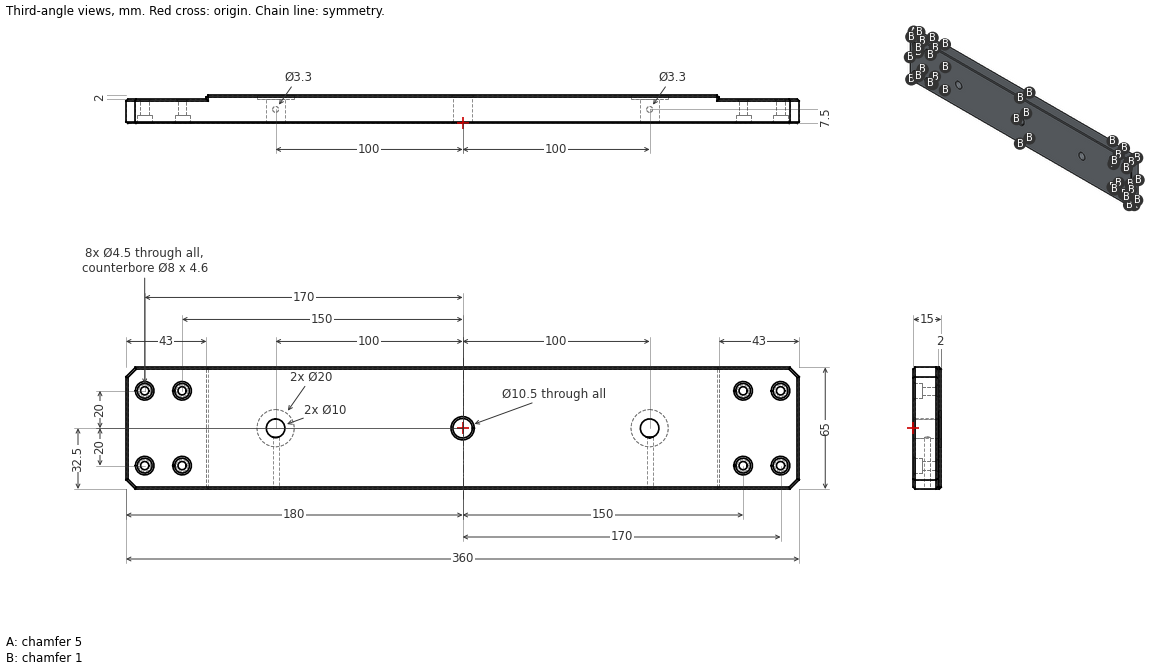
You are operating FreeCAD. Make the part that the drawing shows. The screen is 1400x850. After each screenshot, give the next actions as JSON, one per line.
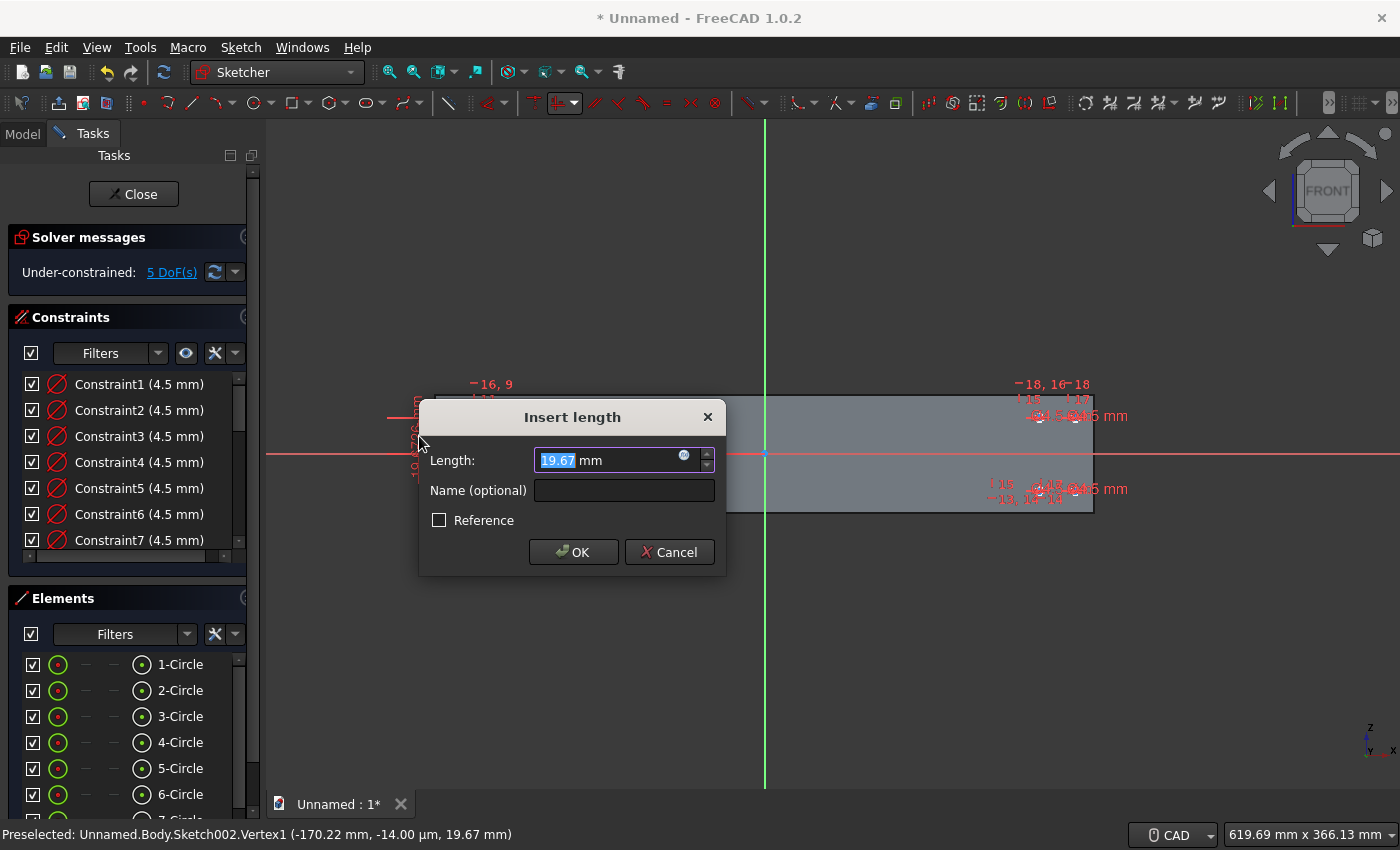
{"action": "type", "text": "20"}
{"action": "key", "text": "Return"}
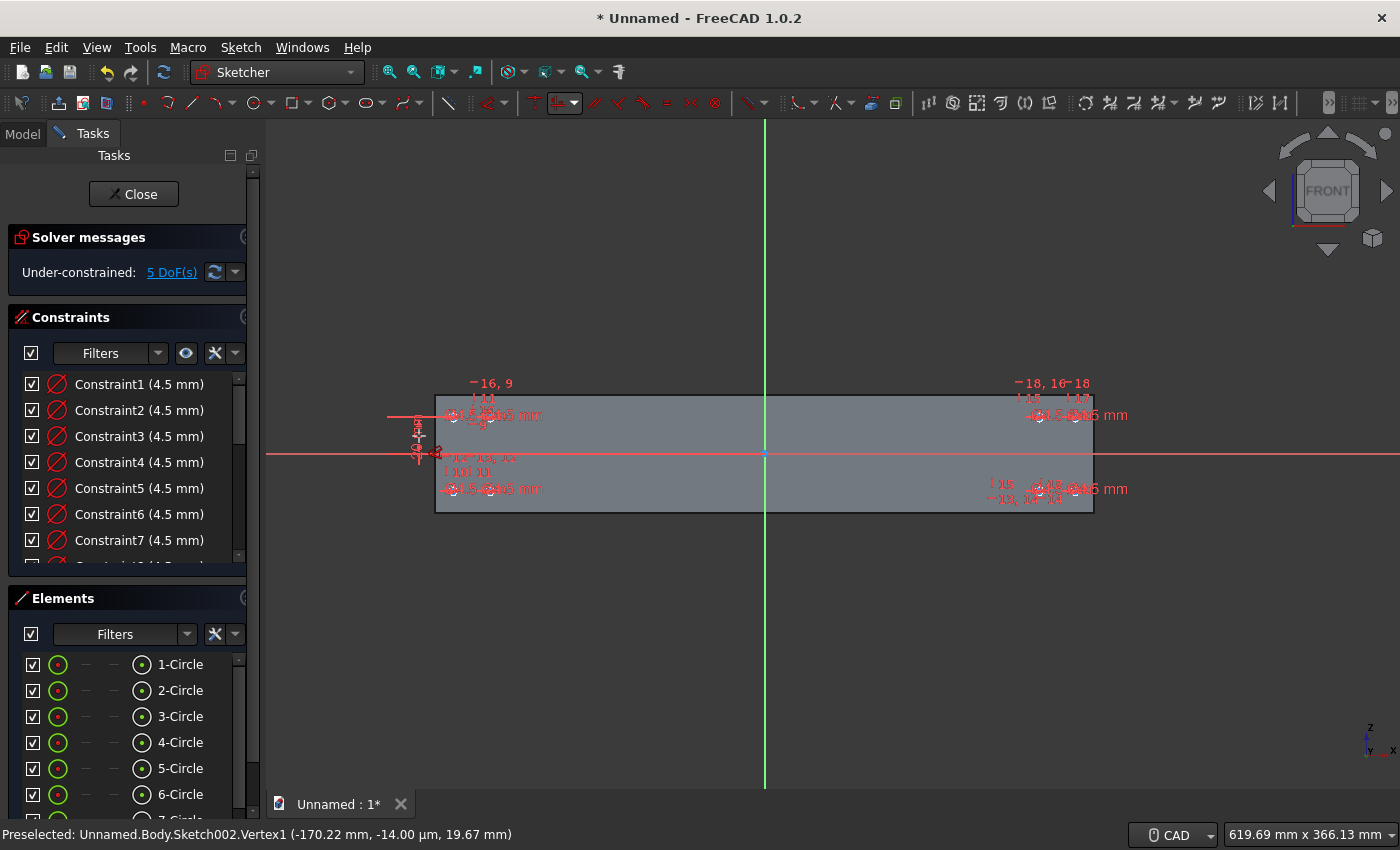
{"action": "left_click", "coordinate": [453, 491]}
{"action": "left_click", "coordinate": [419, 473]}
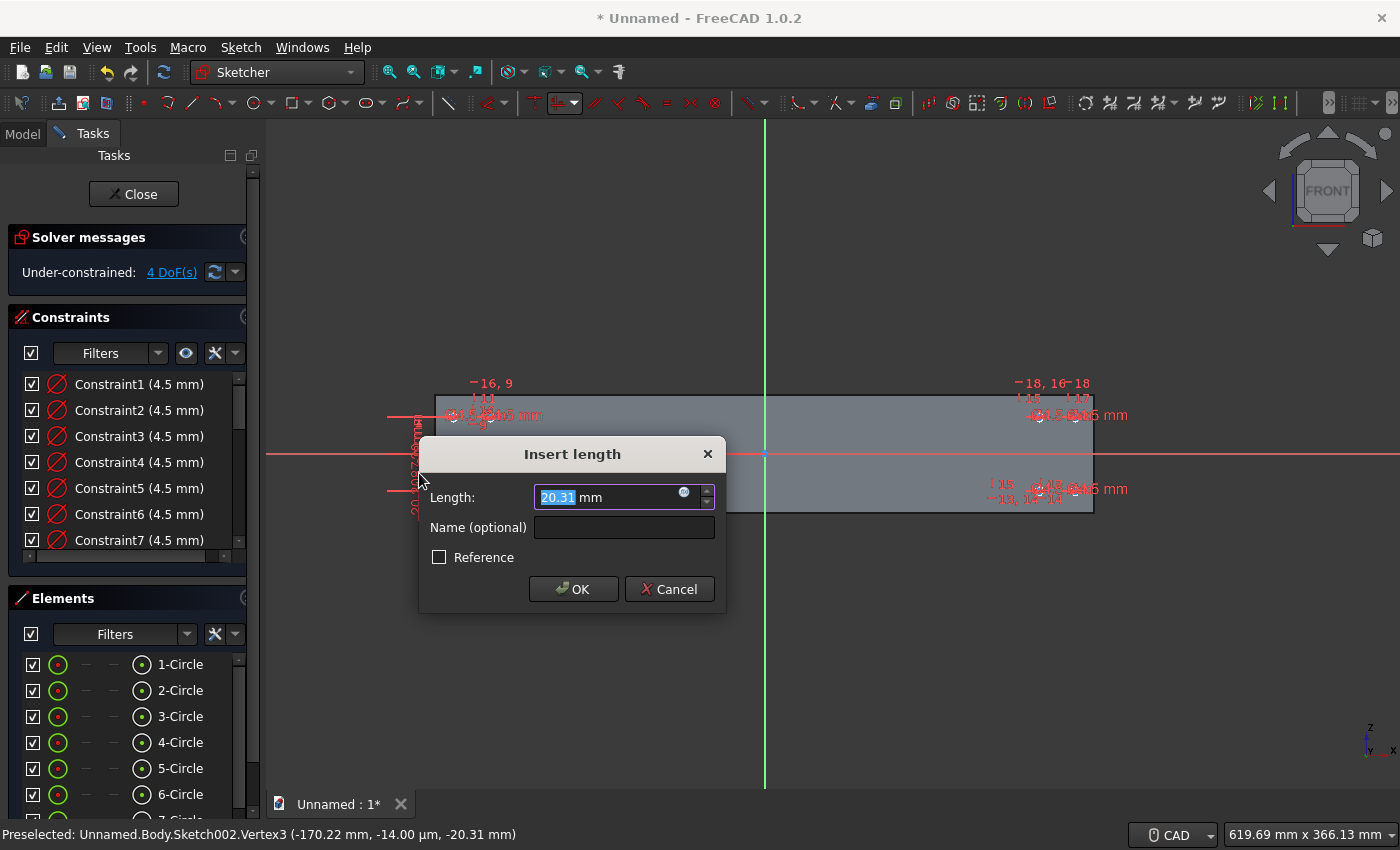
{"action": "type", "text": "20"}
{"action": "key", "text": "Return"}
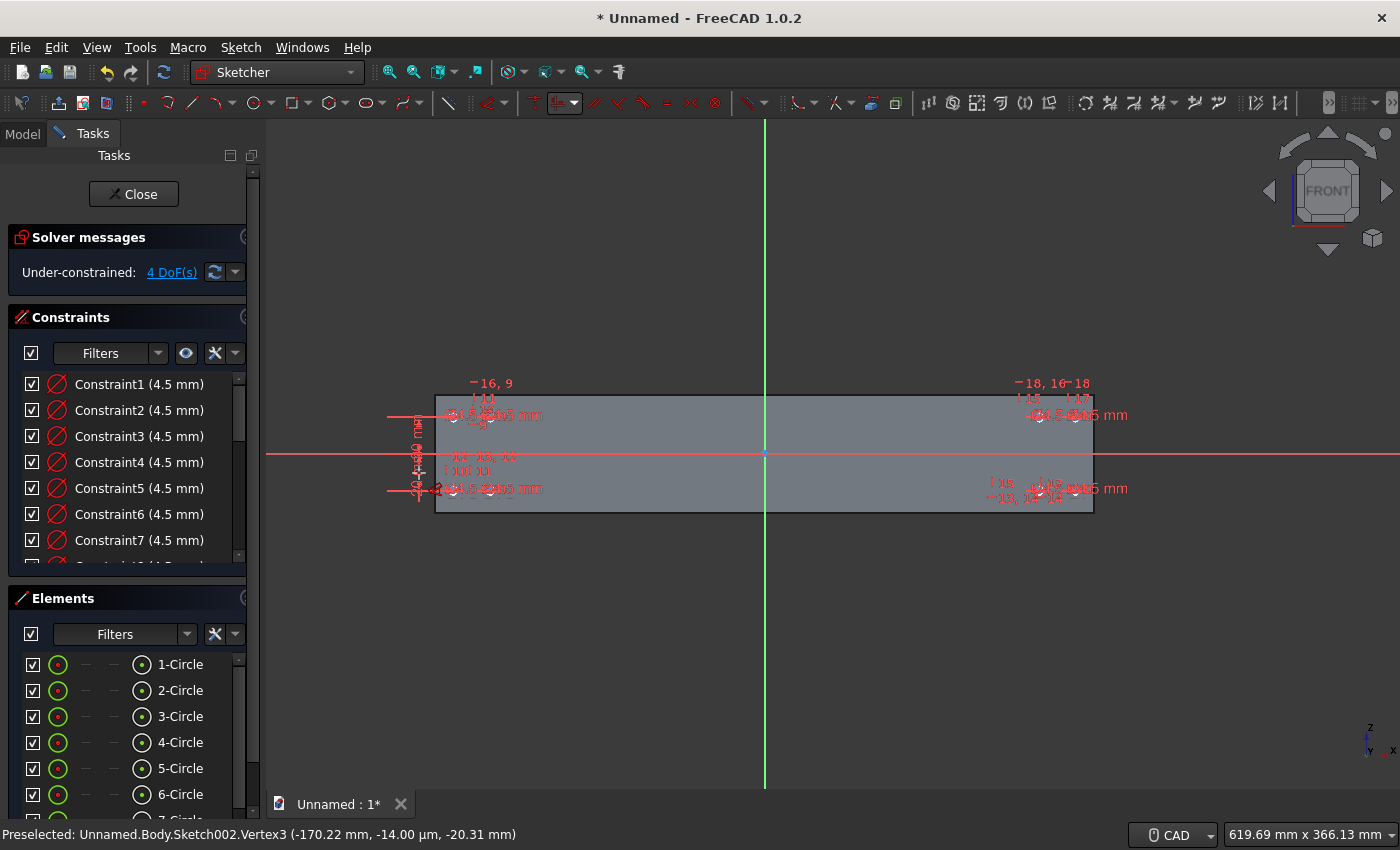
{"action": "left_click", "coordinate": [453, 417]}
{"action": "left_click", "coordinate": [609, 383]}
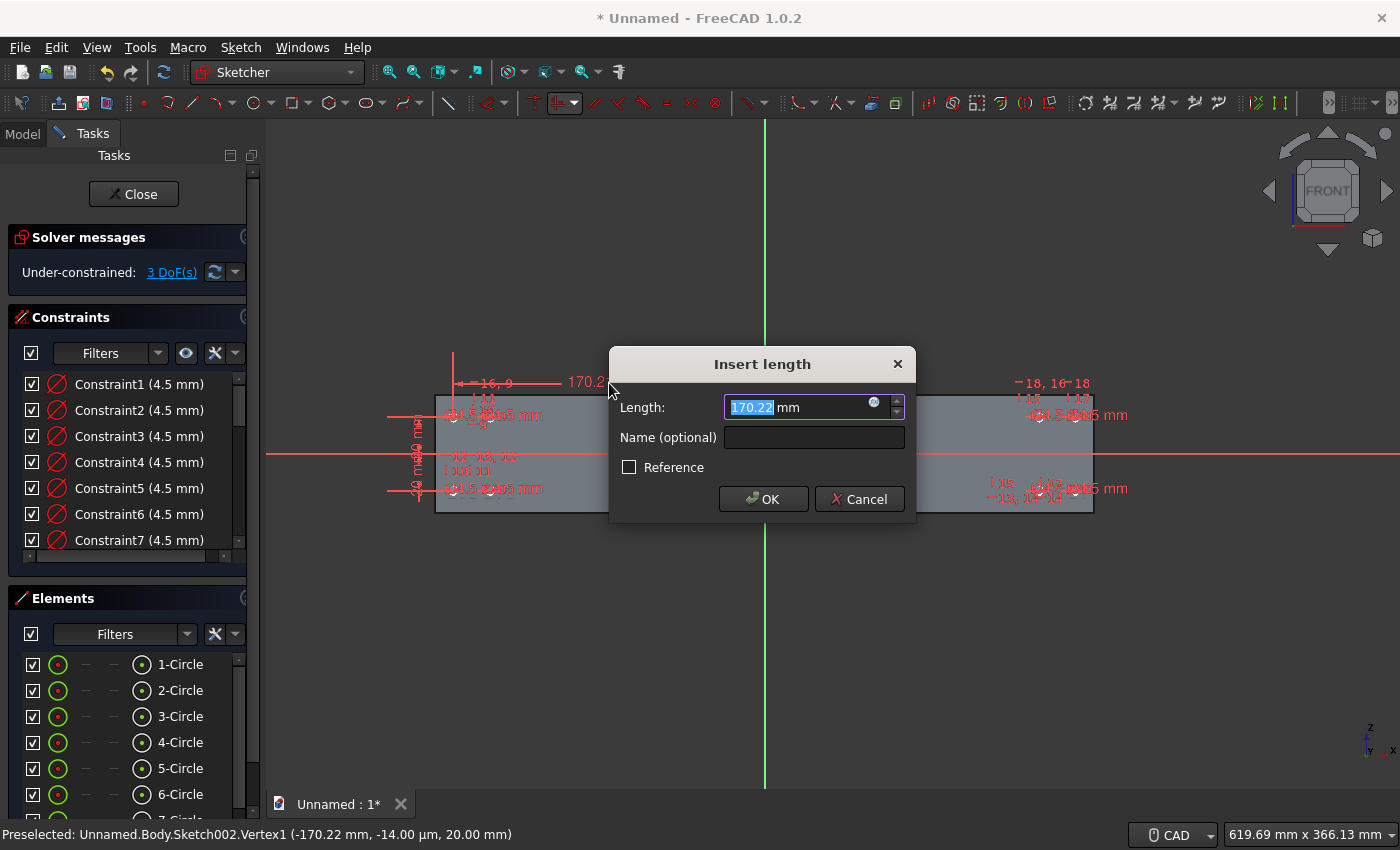
{"action": "type", "text": "170"}
{"action": "key", "text": "Return"}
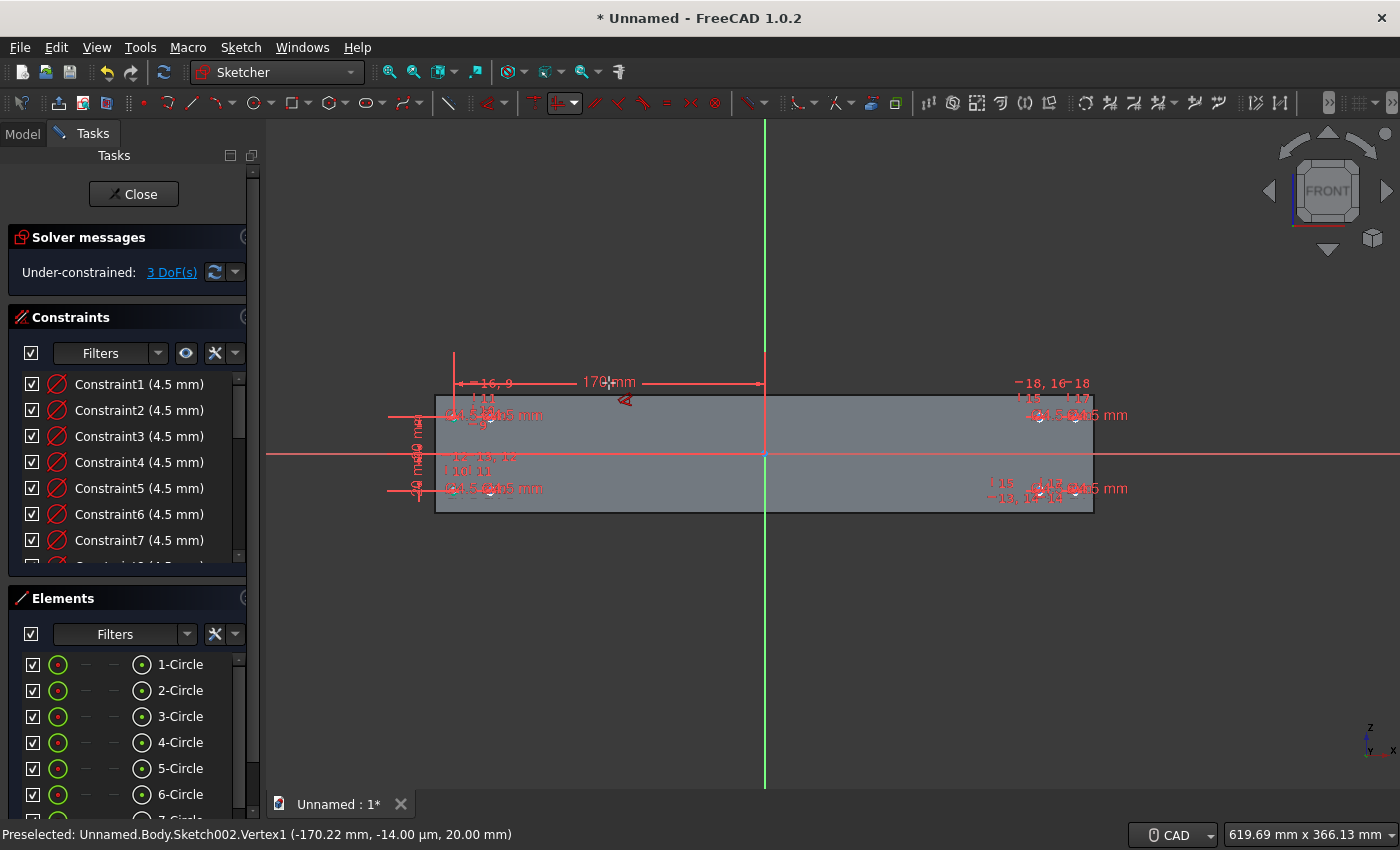
{"action": "left_click", "coordinate": [490, 417]}
{"action": "left_click", "coordinate": [691, 383]}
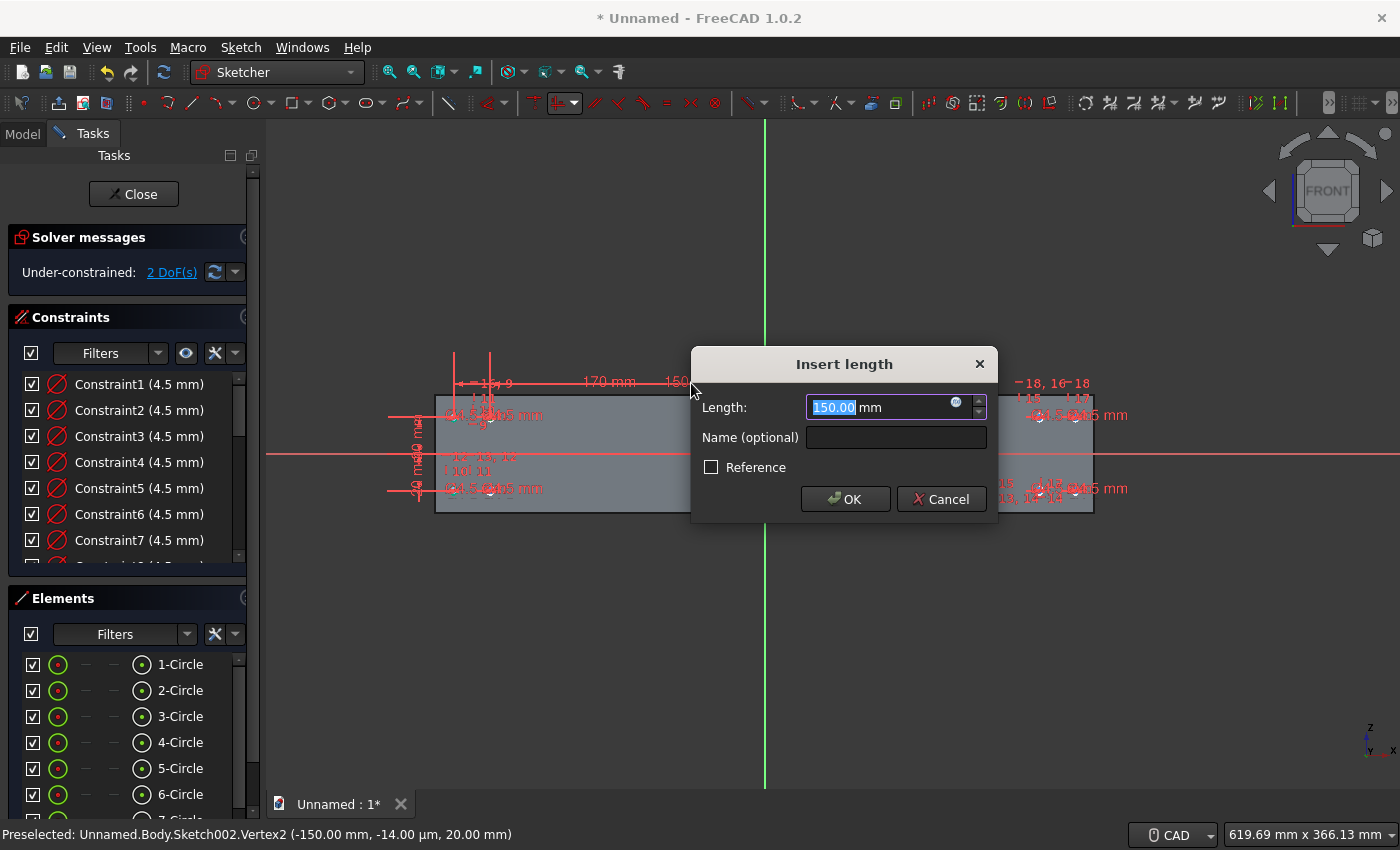
{"action": "type", "text": "150"}
{"action": "key", "text": "Return"}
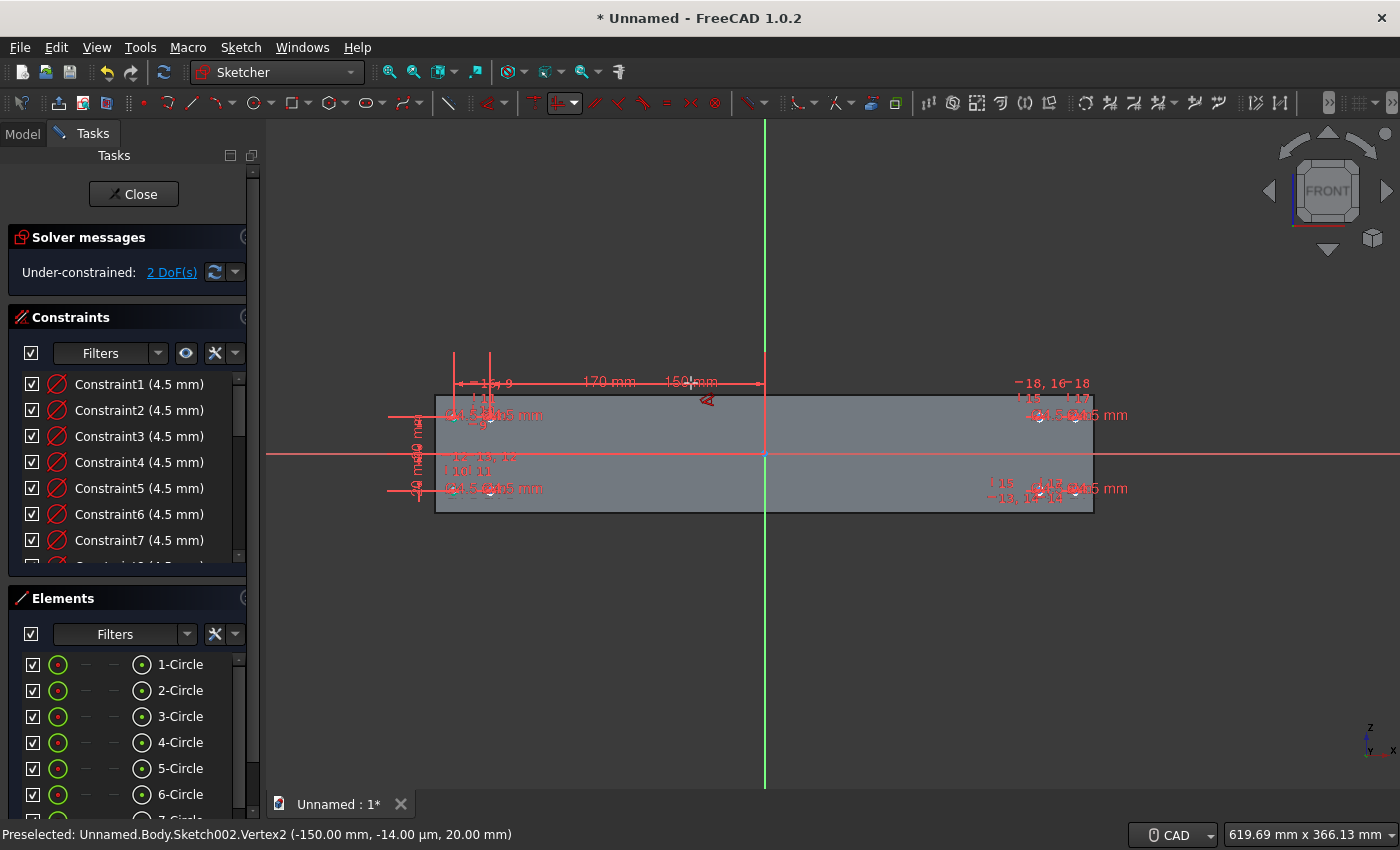
{"action": "left_click", "coordinate": [1039, 491]}
{"action": "left_click", "coordinate": [902, 525]}